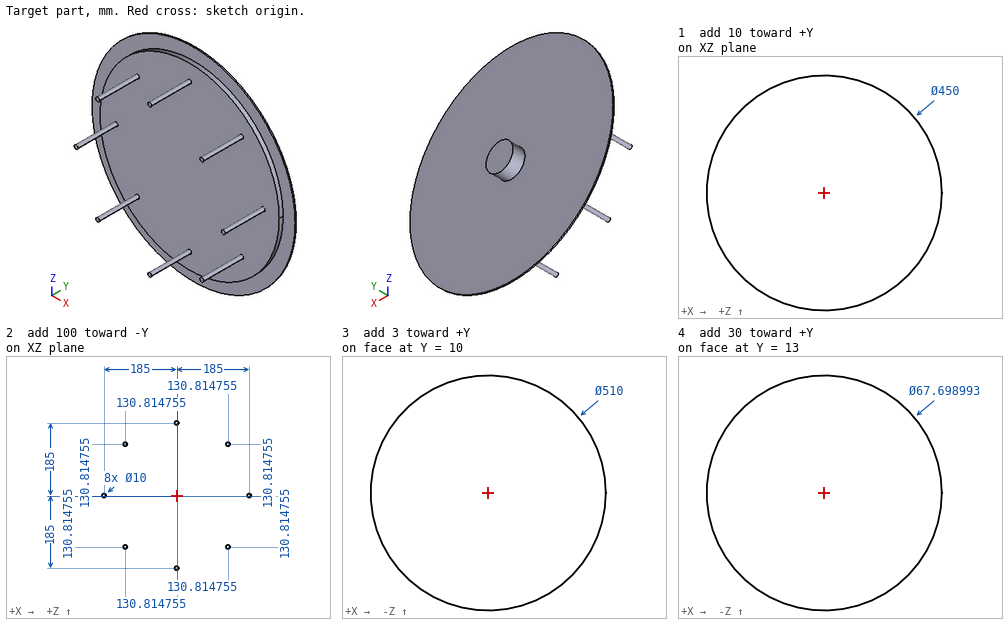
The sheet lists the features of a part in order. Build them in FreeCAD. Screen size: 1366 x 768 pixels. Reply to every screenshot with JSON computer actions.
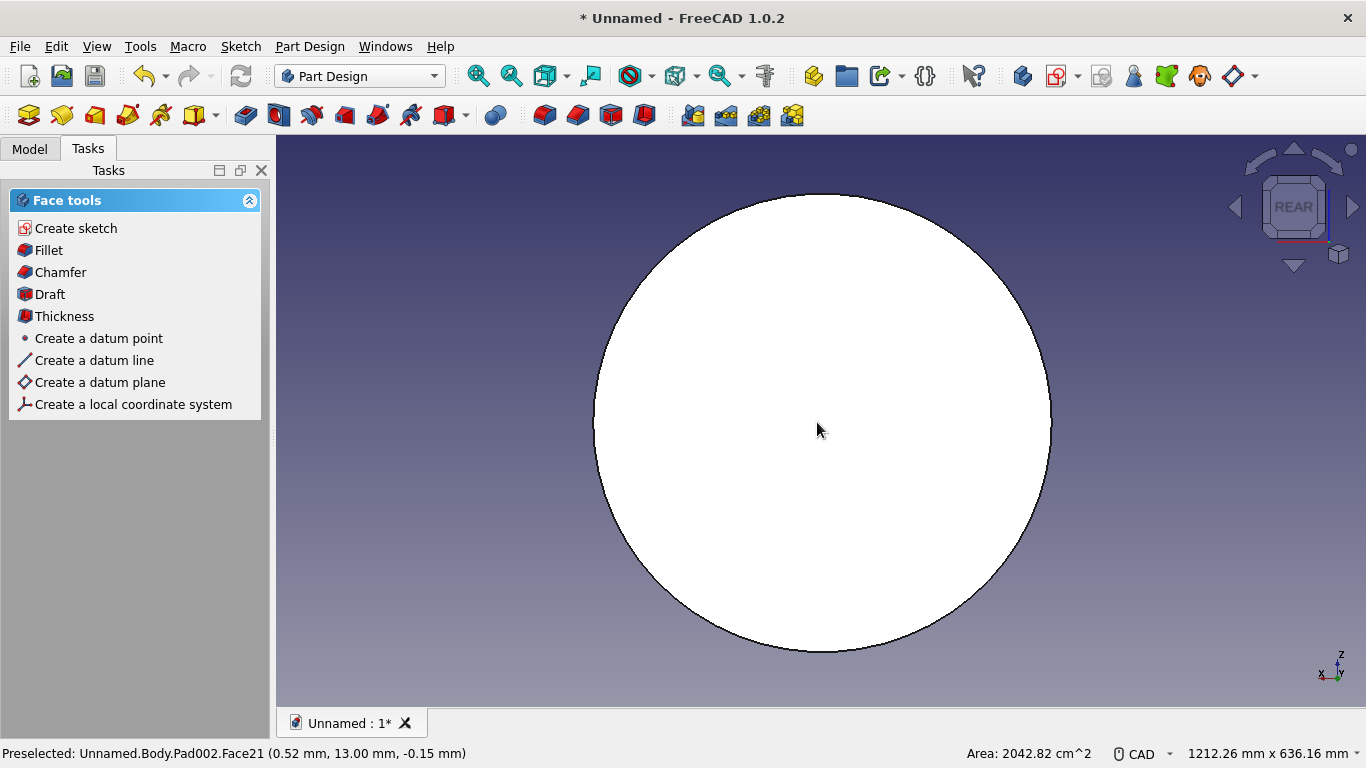
{"action": "left_click", "coordinate": [1056, 76]}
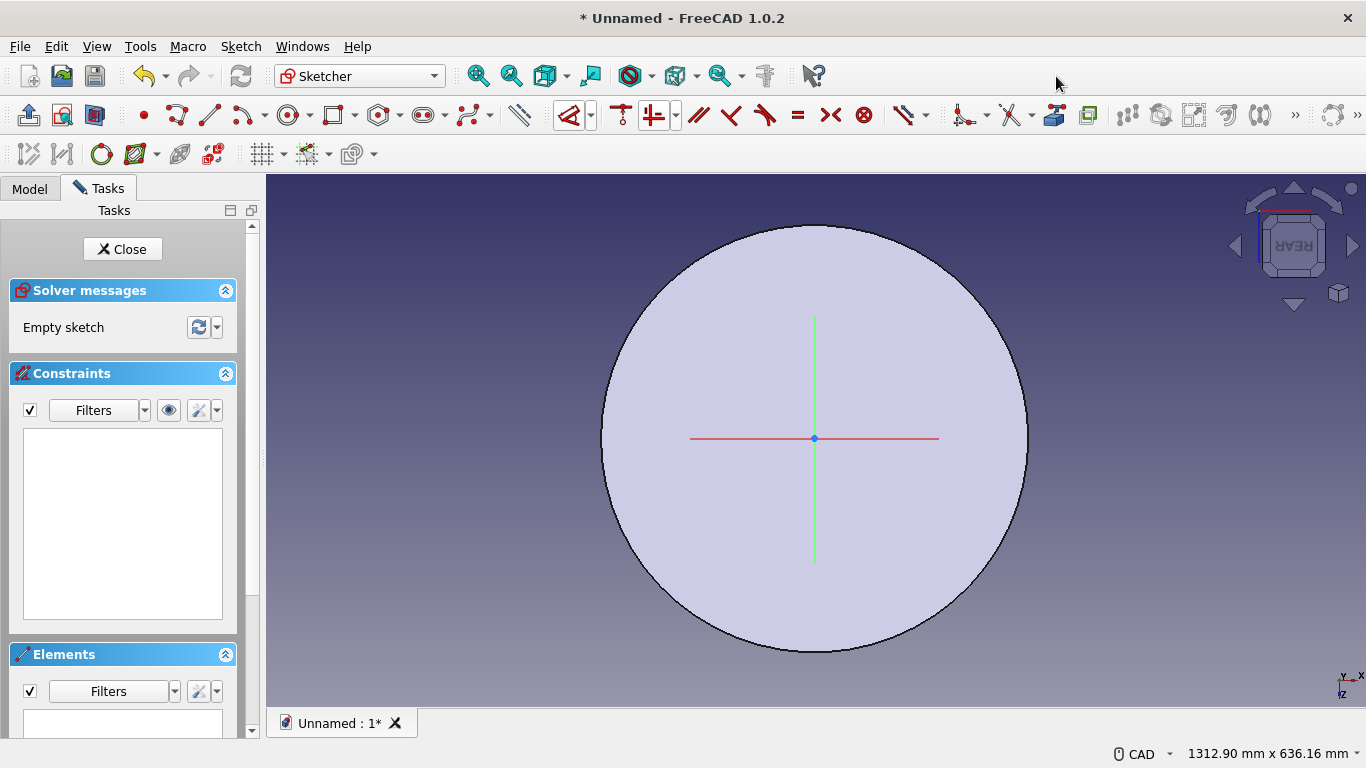
{"action": "scroll", "coordinate": [828, 438], "scroll_direction": "up", "scroll_amount": 9}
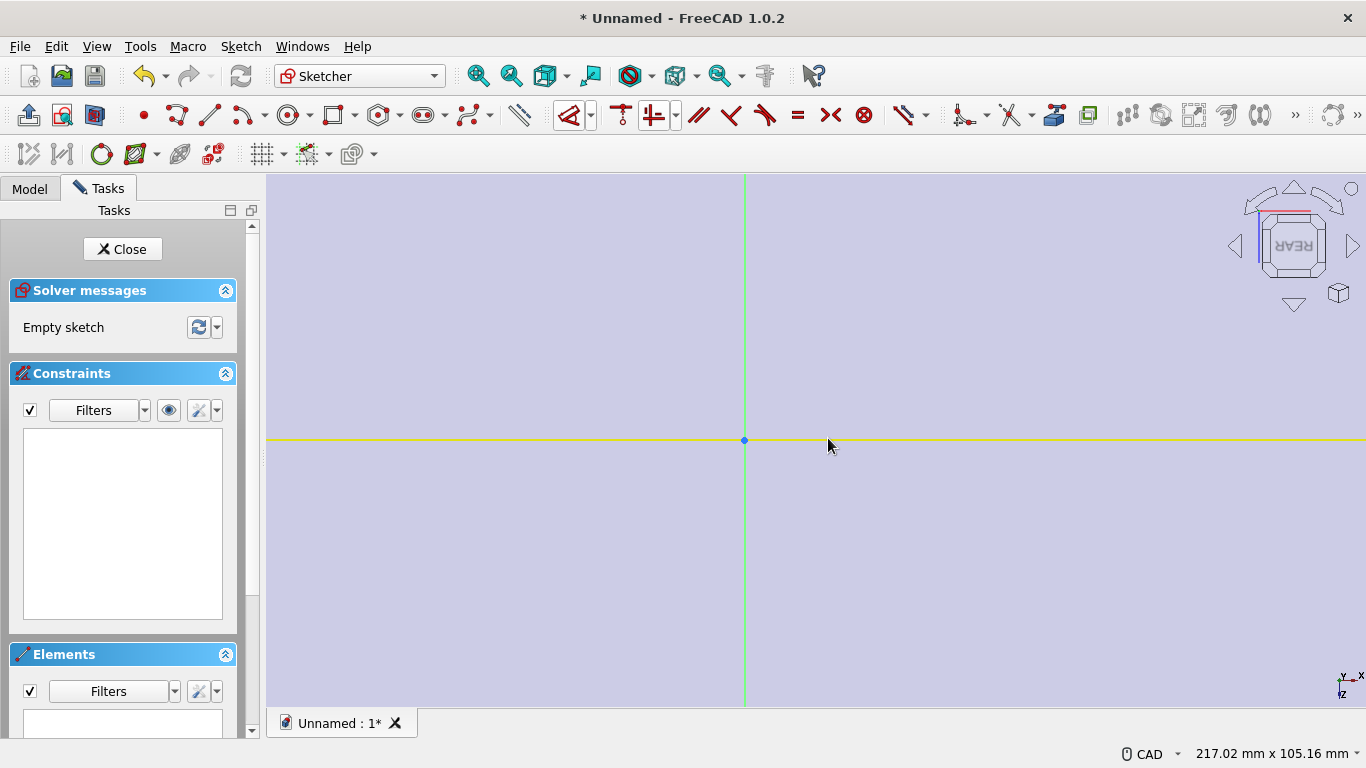
{"action": "key", "text": "g c"}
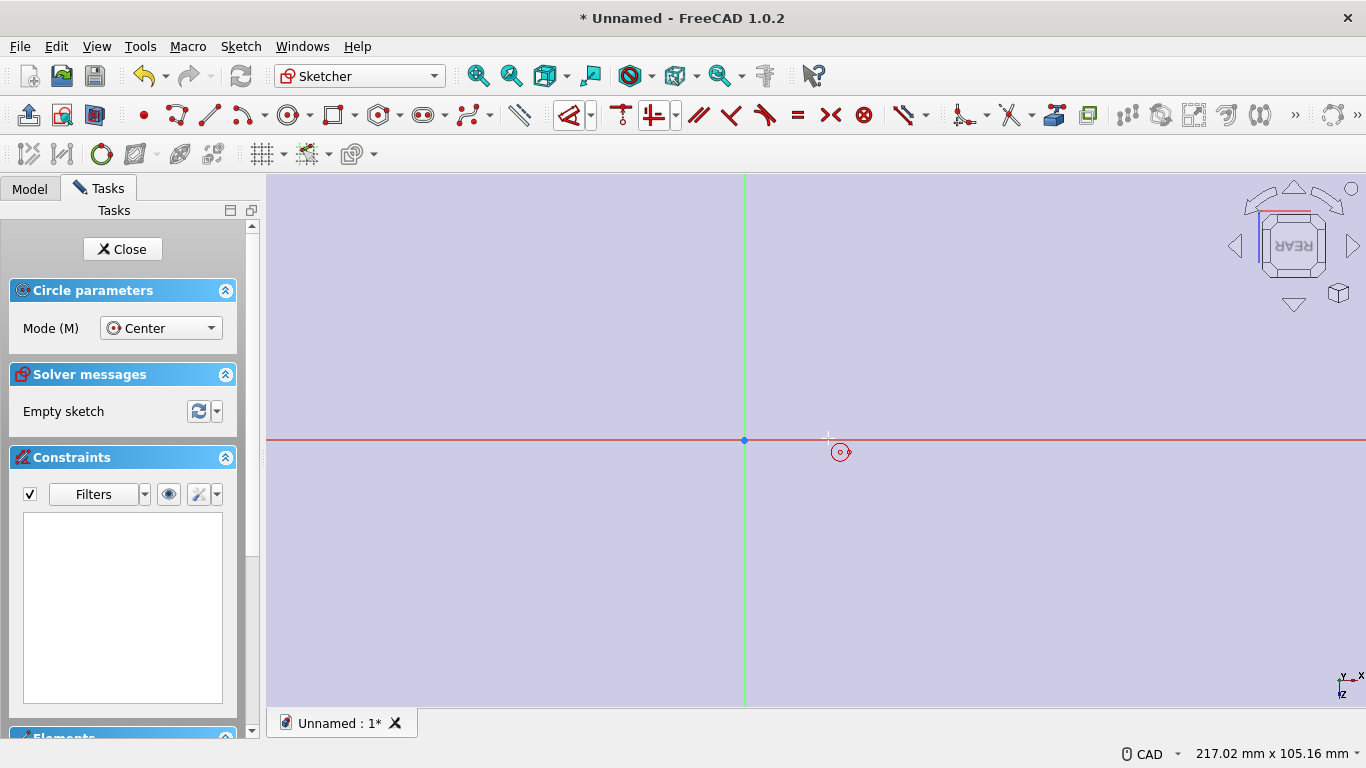
{"action": "left_click", "coordinate": [745, 440]}
{"action": "left_click", "coordinate": [866, 319]}
{"action": "key", "text": "Escape"}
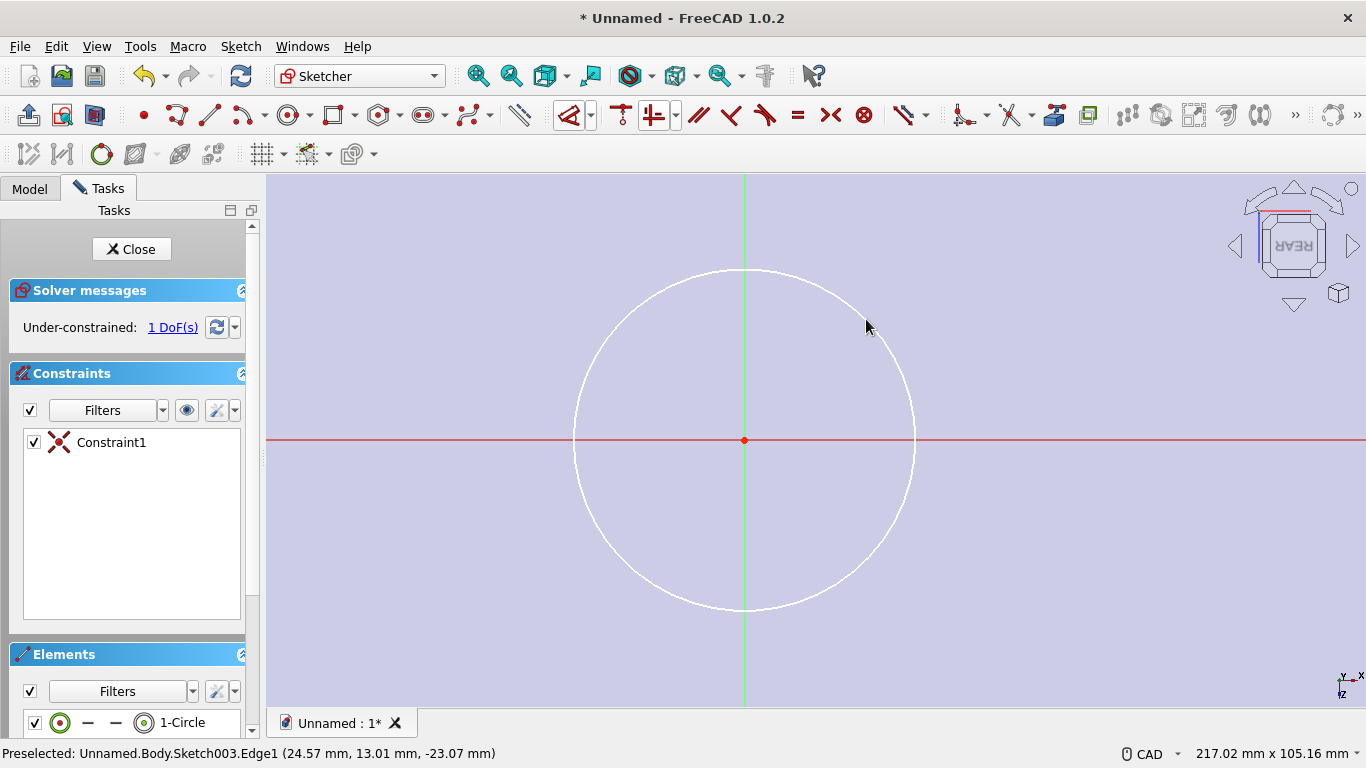
{"action": "left_click", "coordinate": [865, 319]}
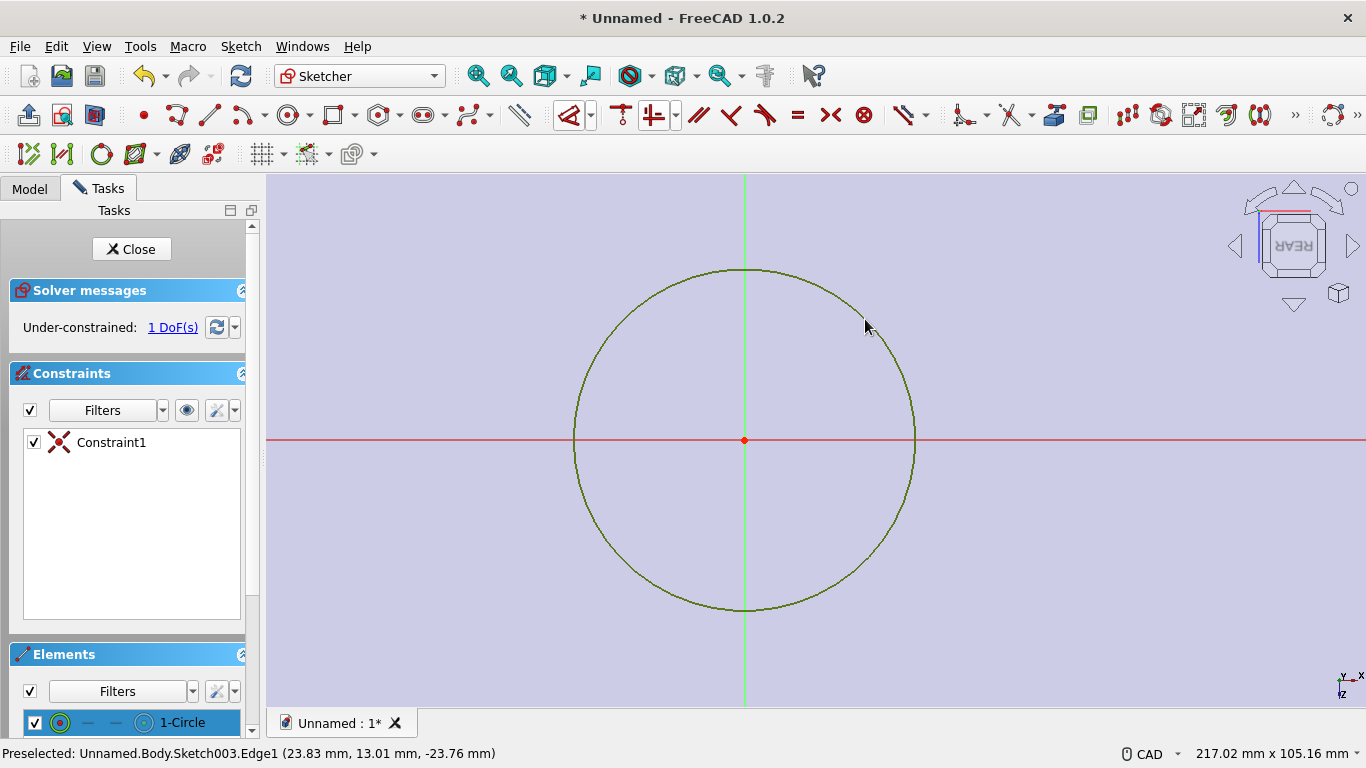
{"action": "left_click", "coordinate": [590, 116]}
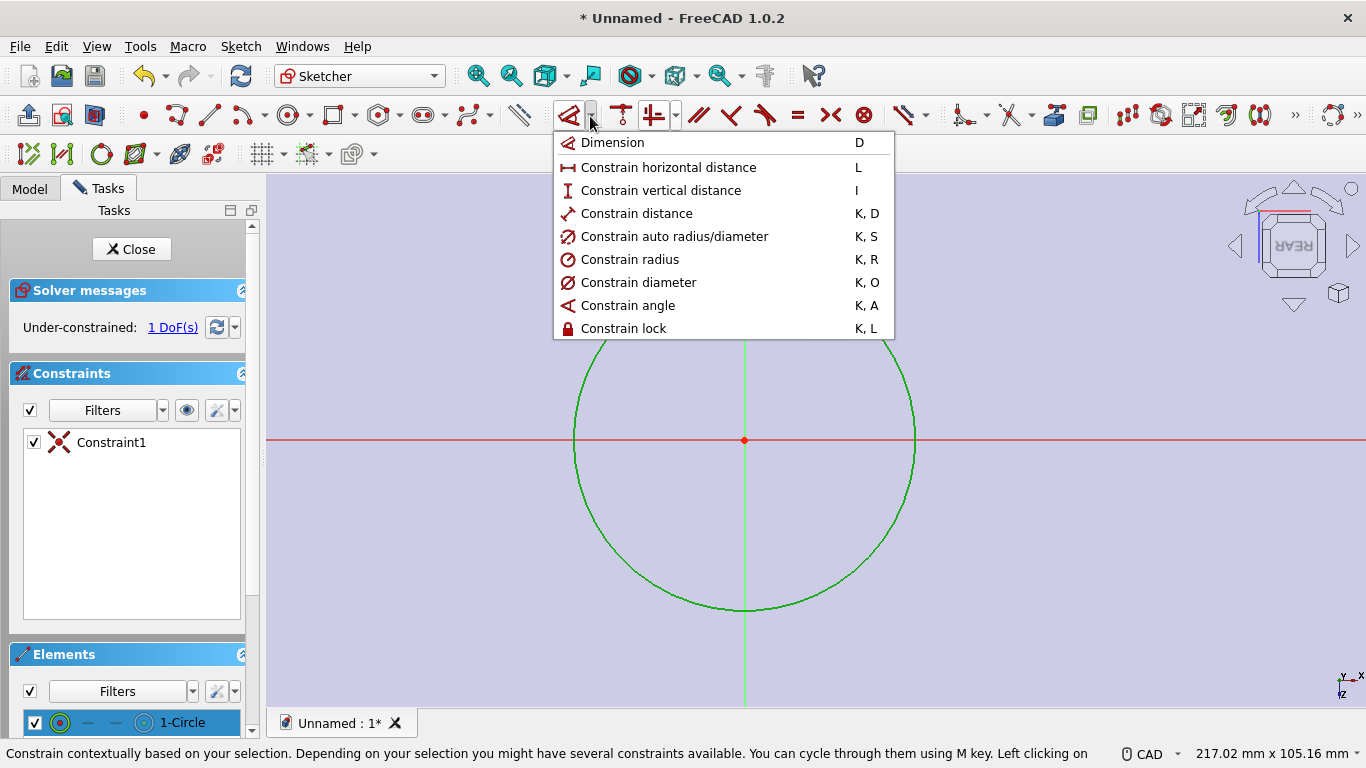
{"action": "left_click", "coordinate": [724, 282]}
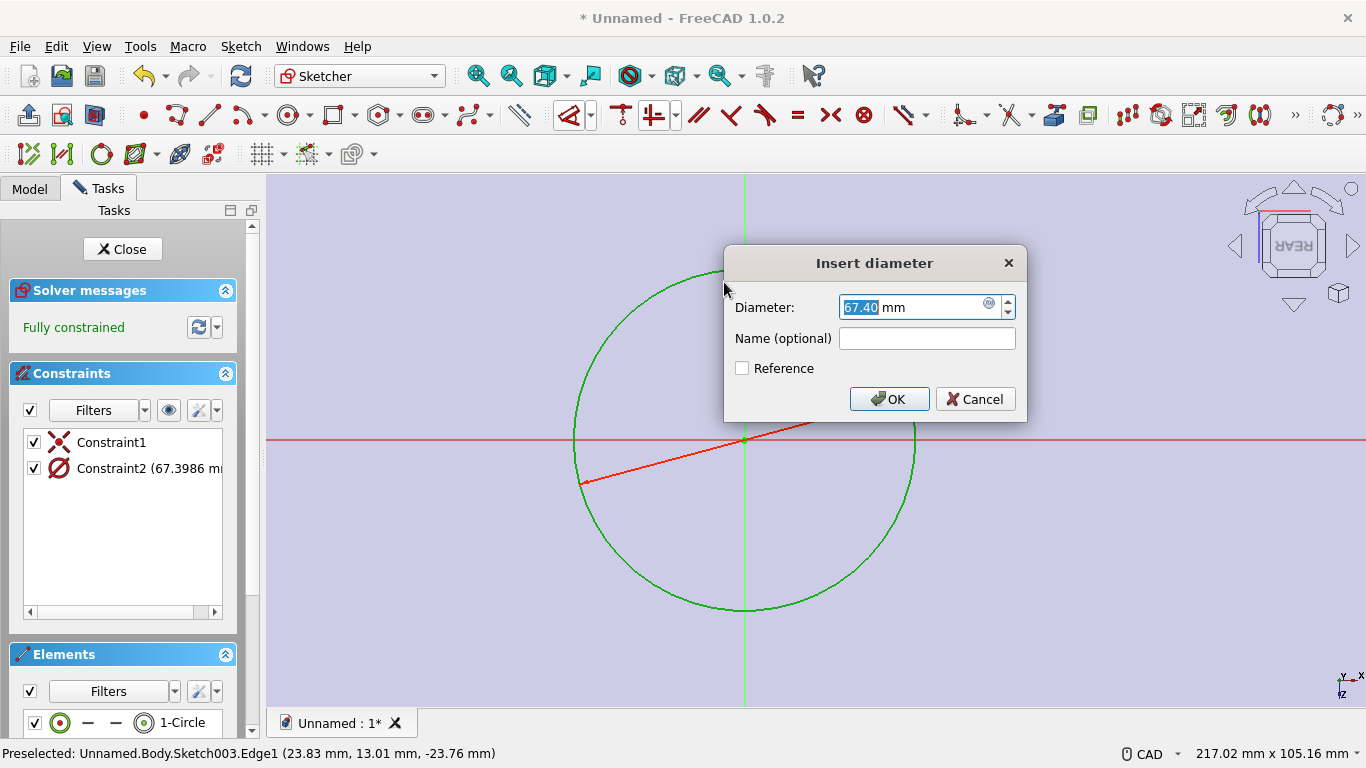
{"action": "type", "text": "67.698993"}
{"action": "key", "text": "Return"}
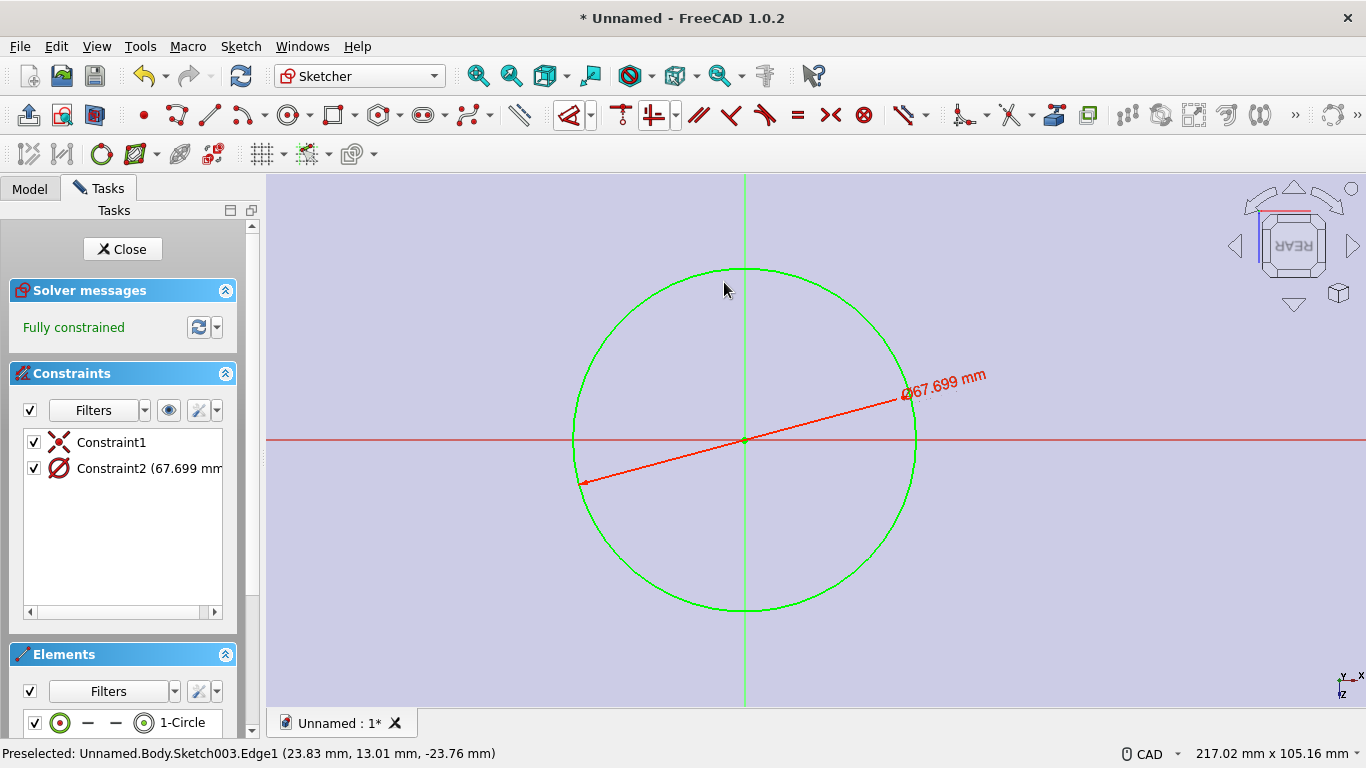
{"action": "left_click", "coordinate": [123, 249]}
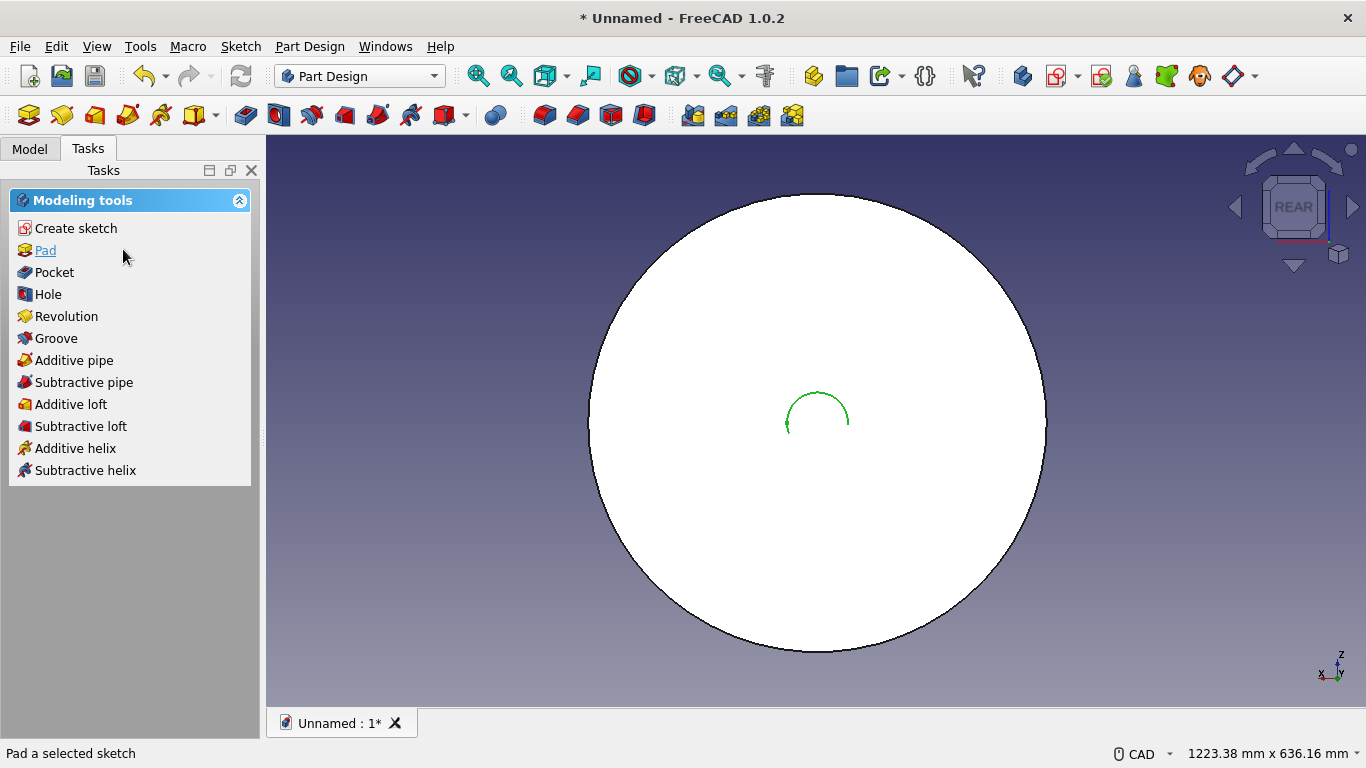
{"action": "left_click", "coordinate": [29, 116]}